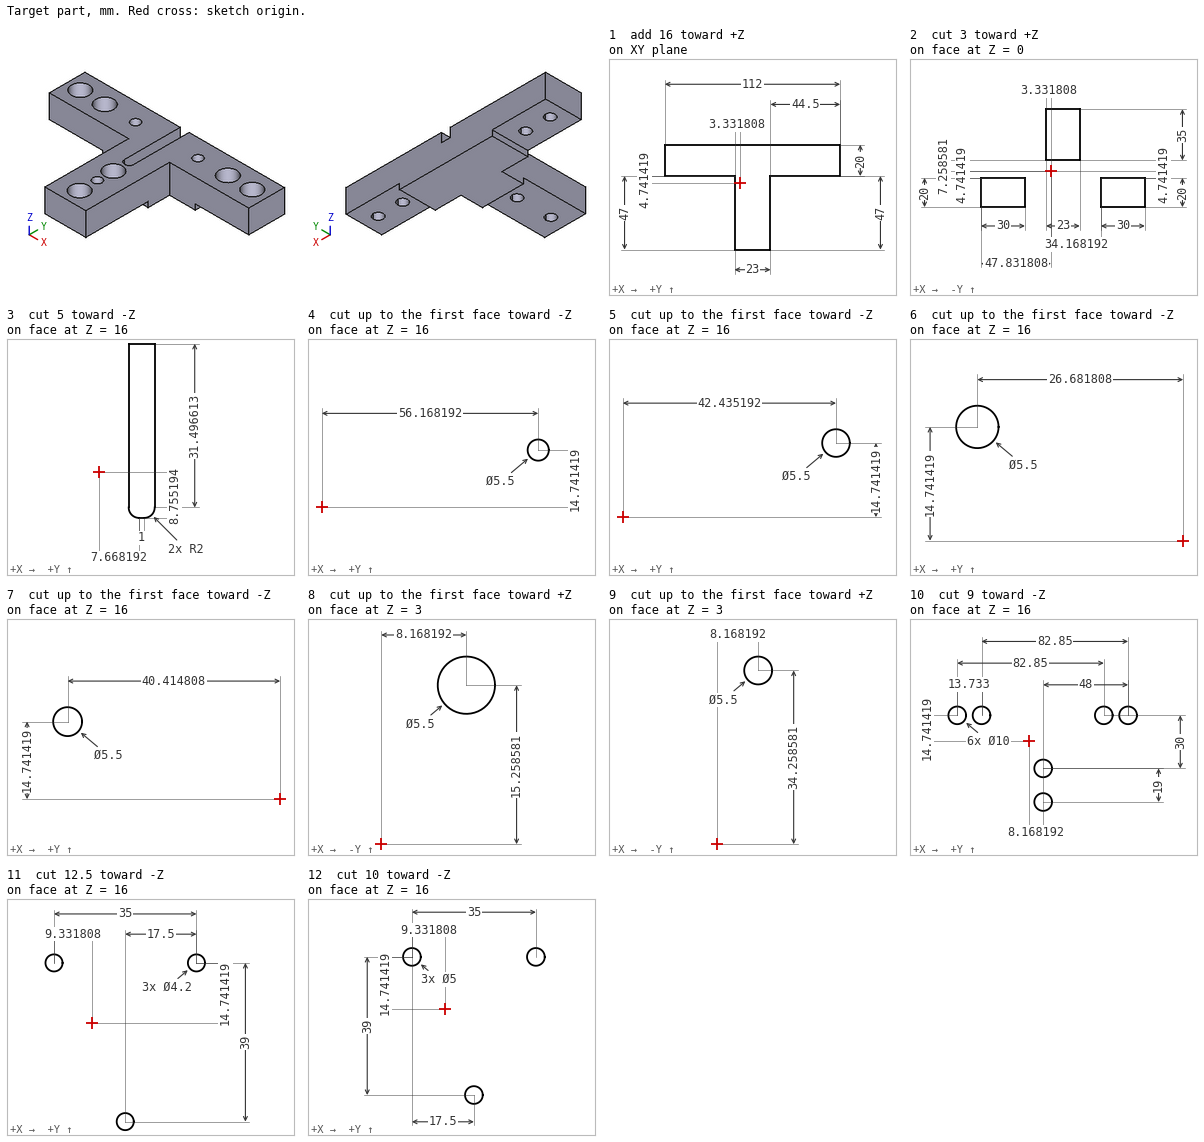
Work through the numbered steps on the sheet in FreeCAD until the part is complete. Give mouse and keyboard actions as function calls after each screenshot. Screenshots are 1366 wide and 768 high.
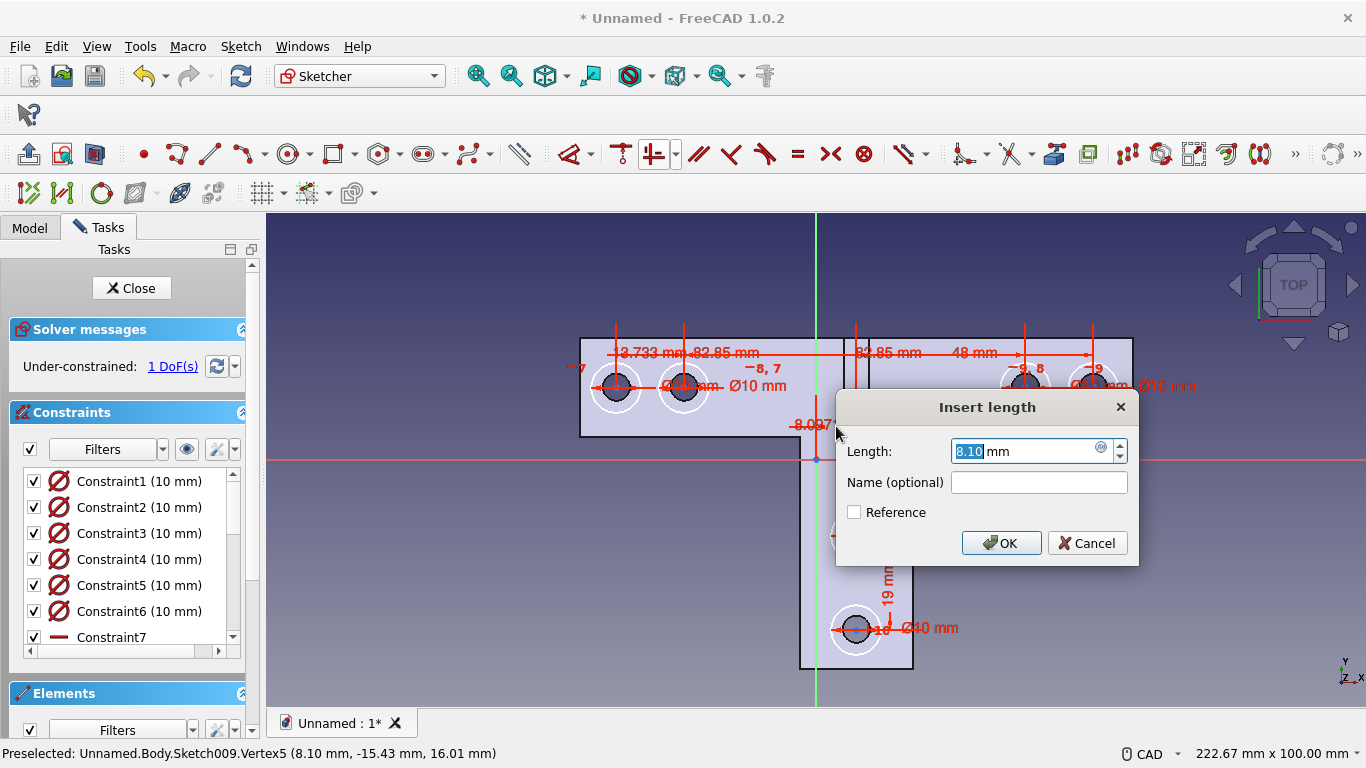
text(8.168192)
key(Return)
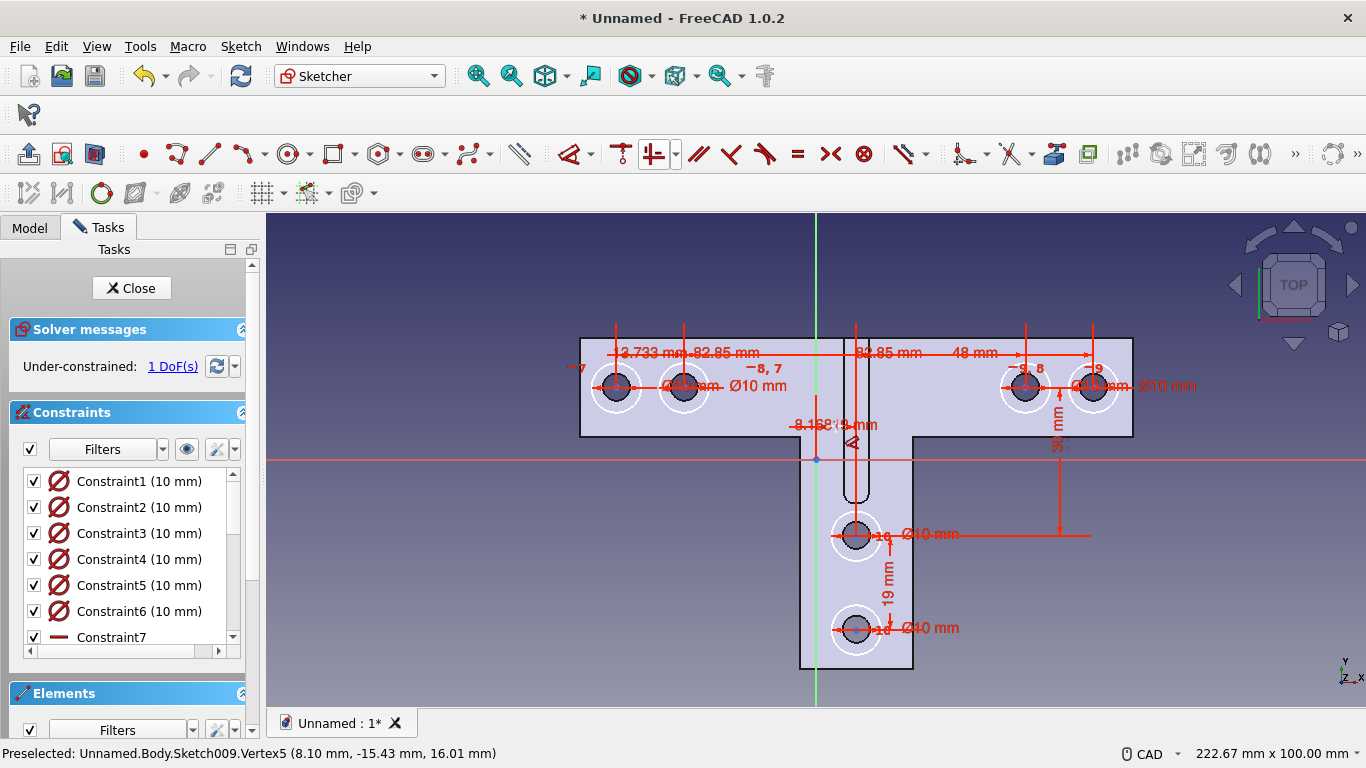
click(616, 388)
click(582, 424)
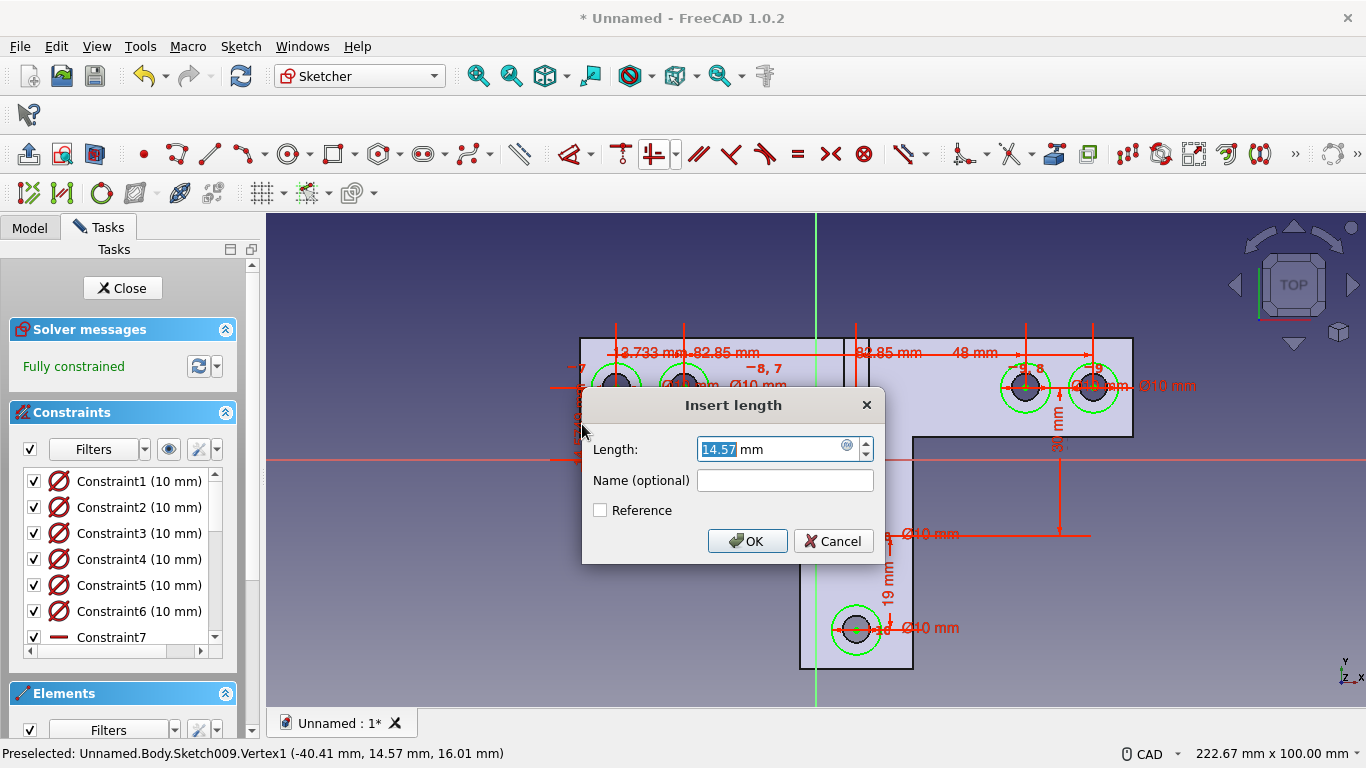
text(14.741419)
key(Return)
key(Escape)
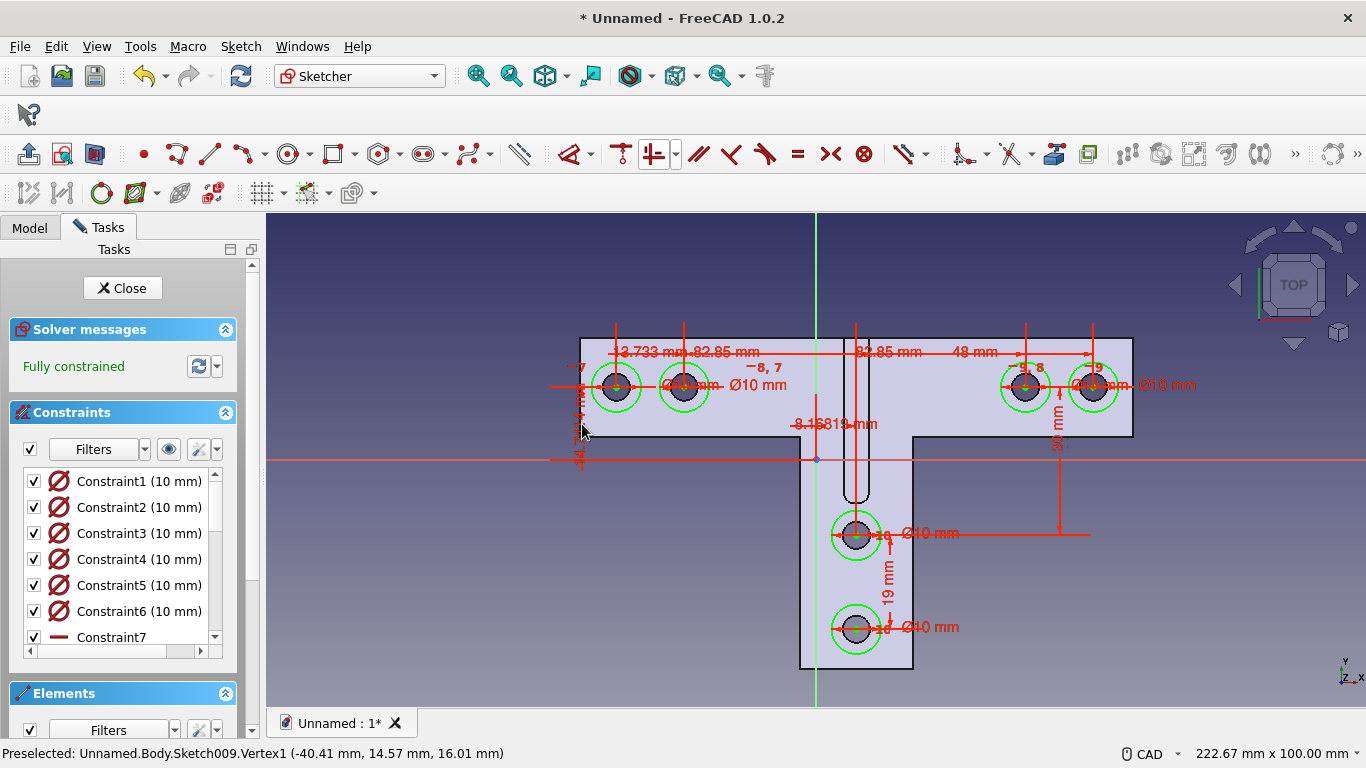
click(123, 288)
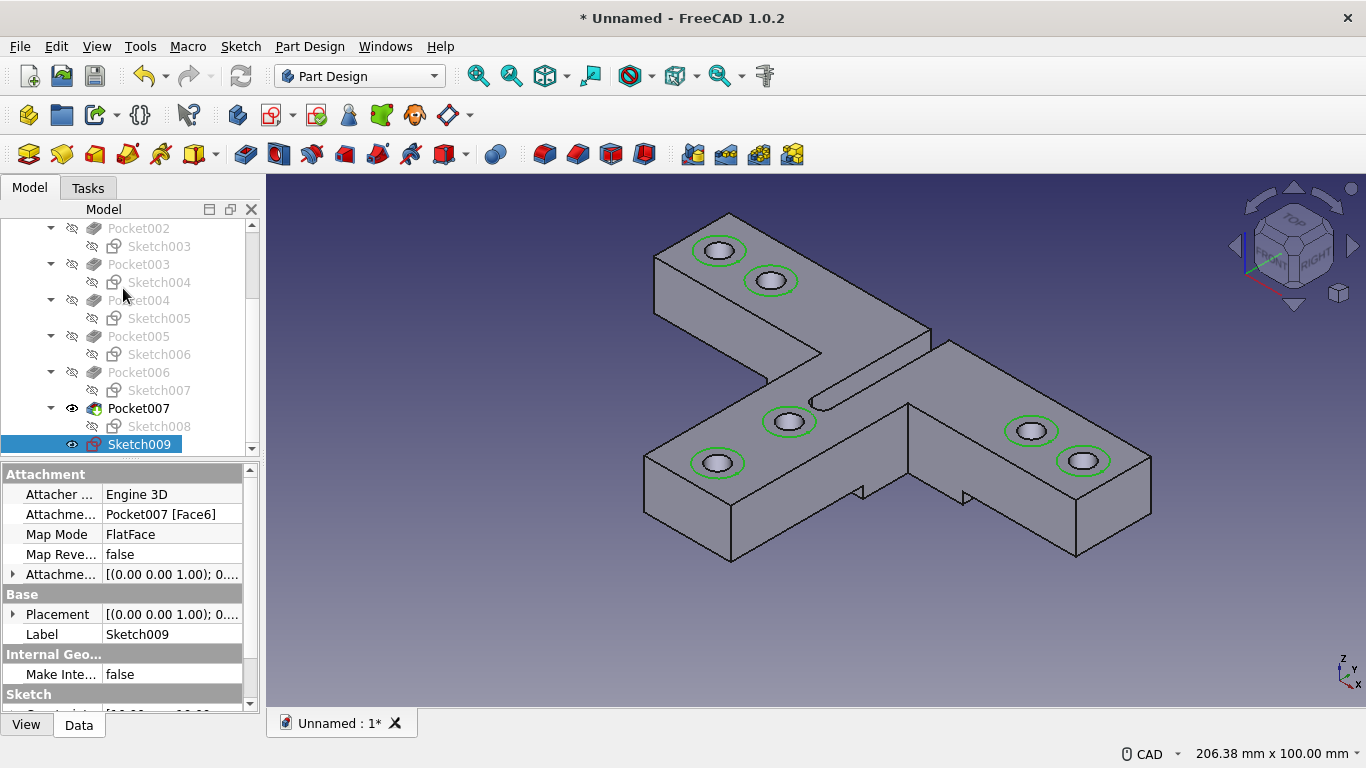
click(246, 154)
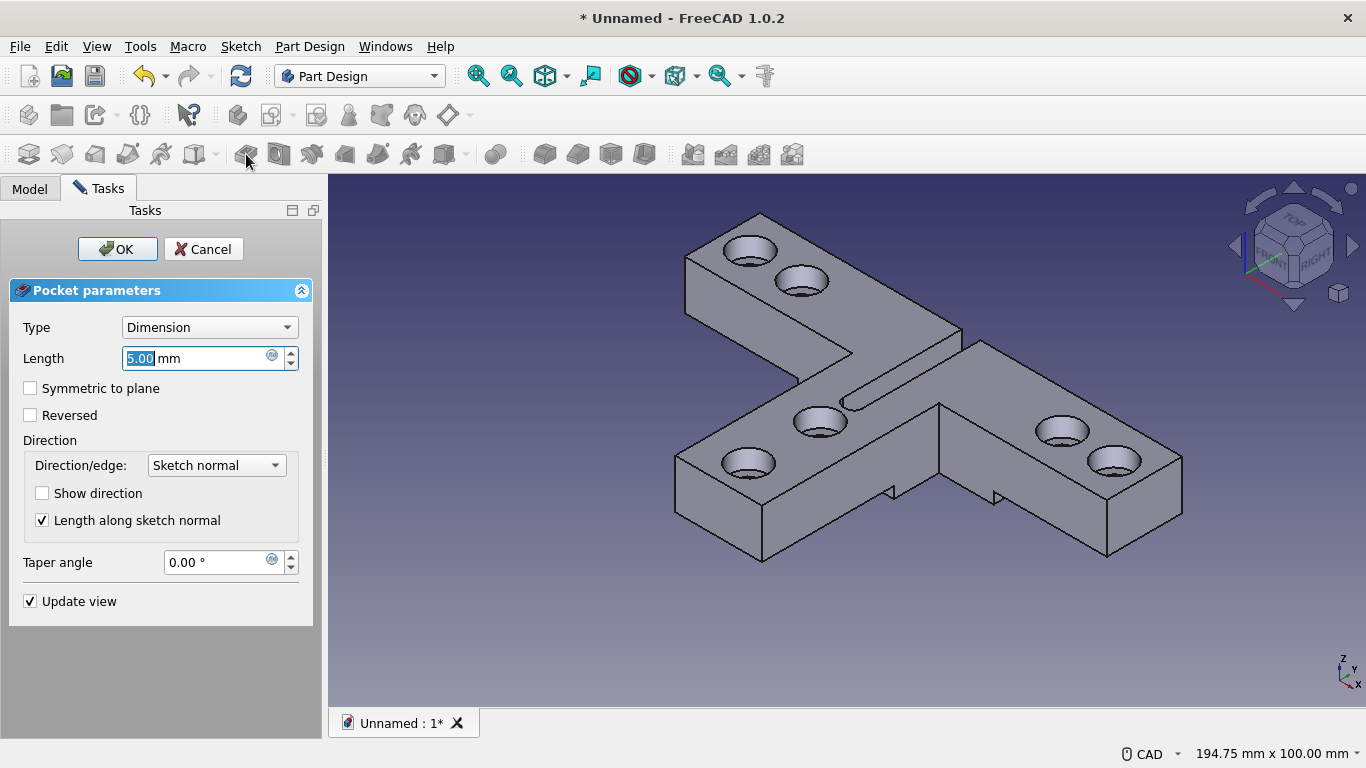
text(9)
key(Tab)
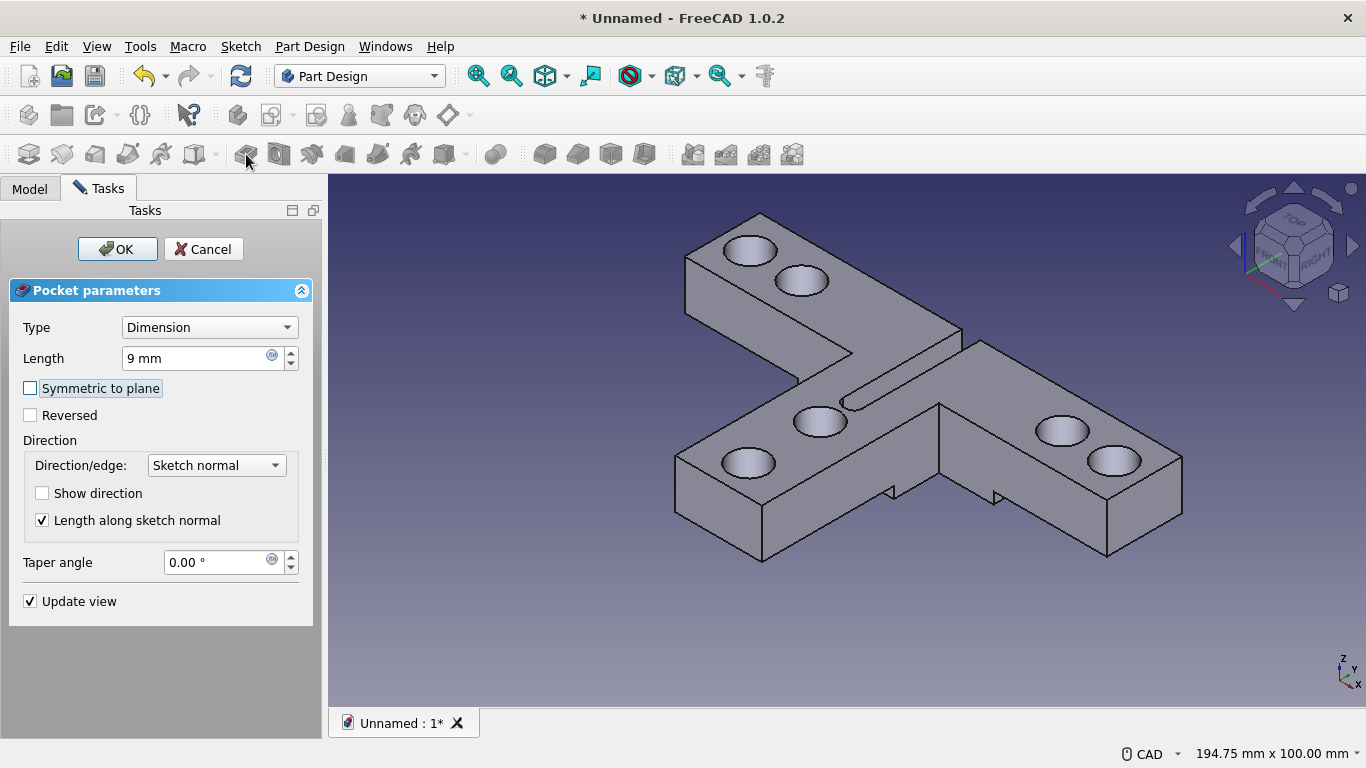
click(118, 249)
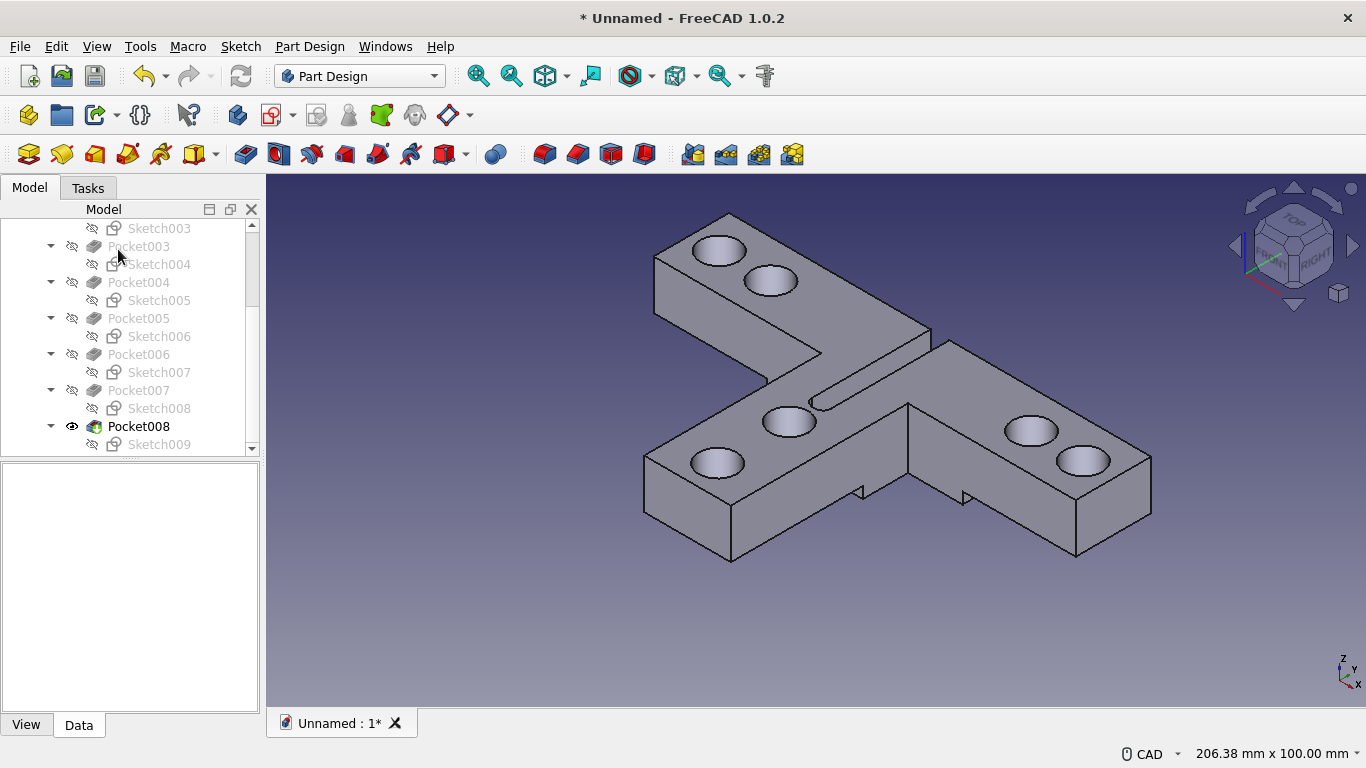
click(826, 330)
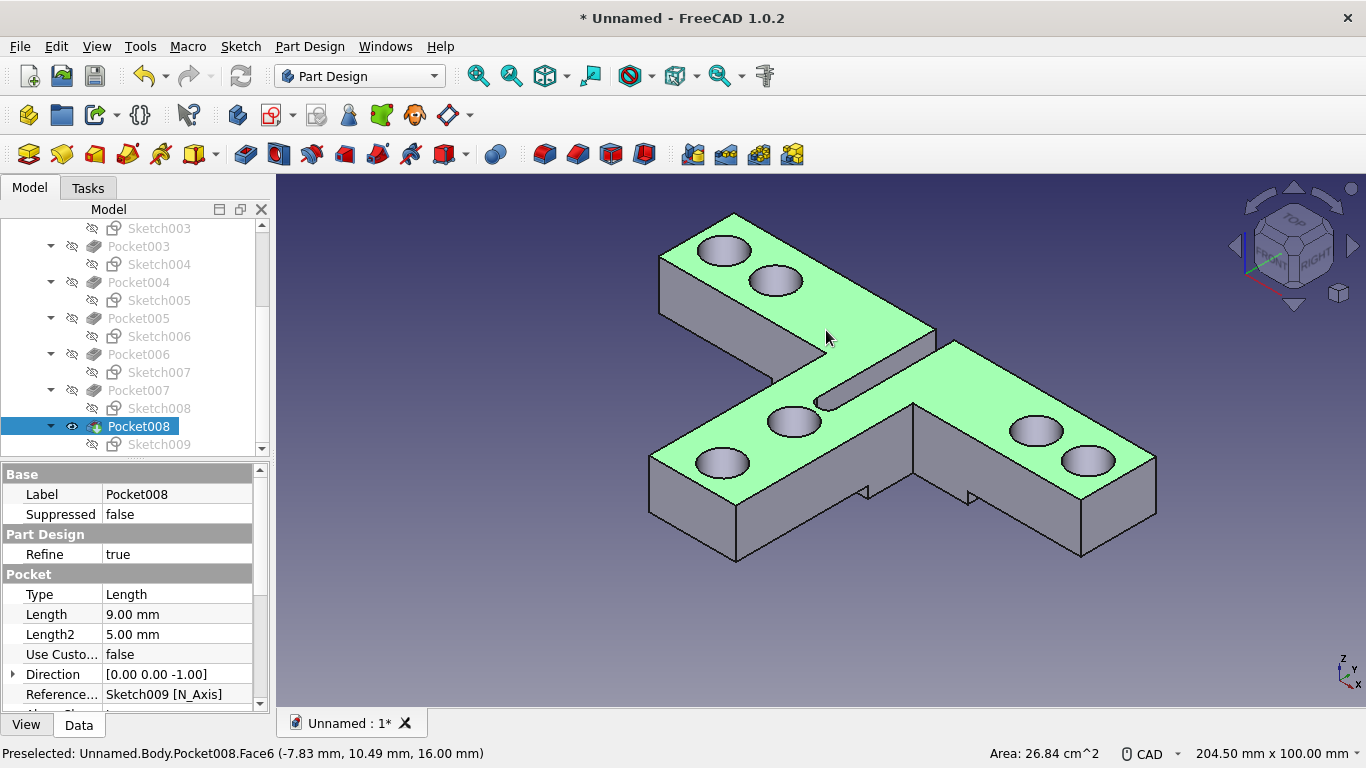
click(270, 116)